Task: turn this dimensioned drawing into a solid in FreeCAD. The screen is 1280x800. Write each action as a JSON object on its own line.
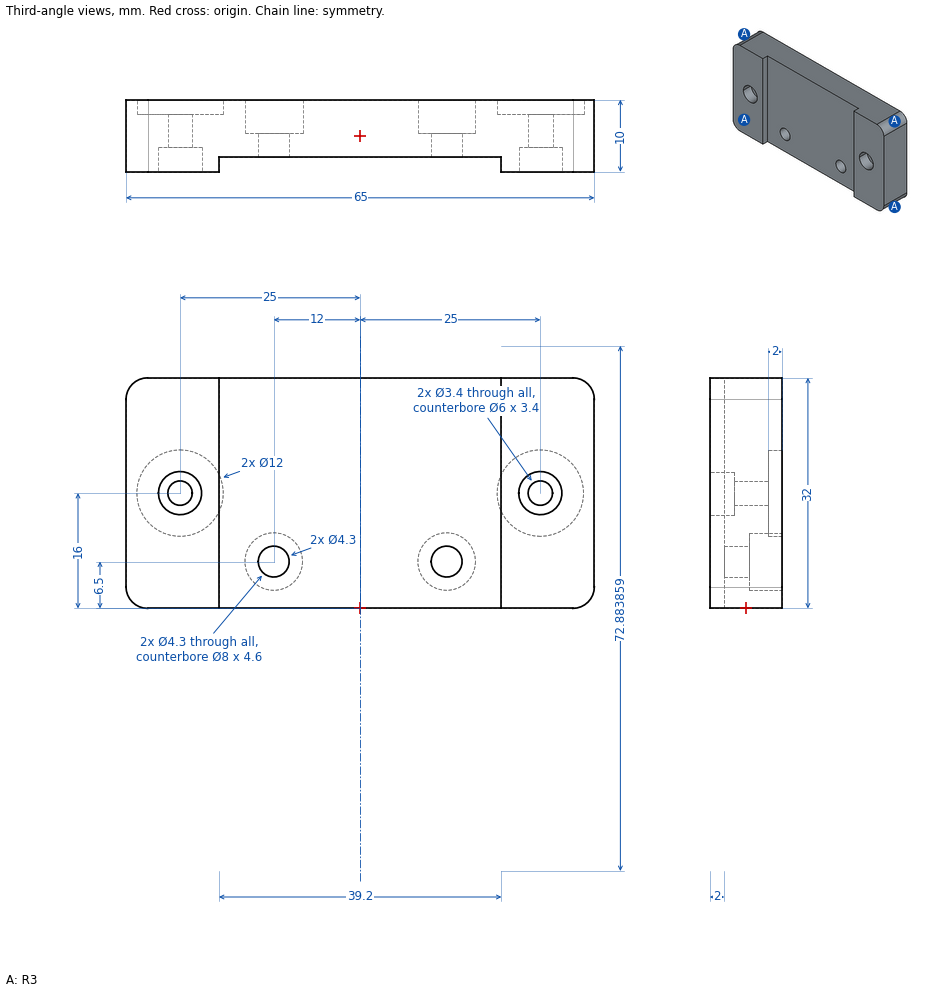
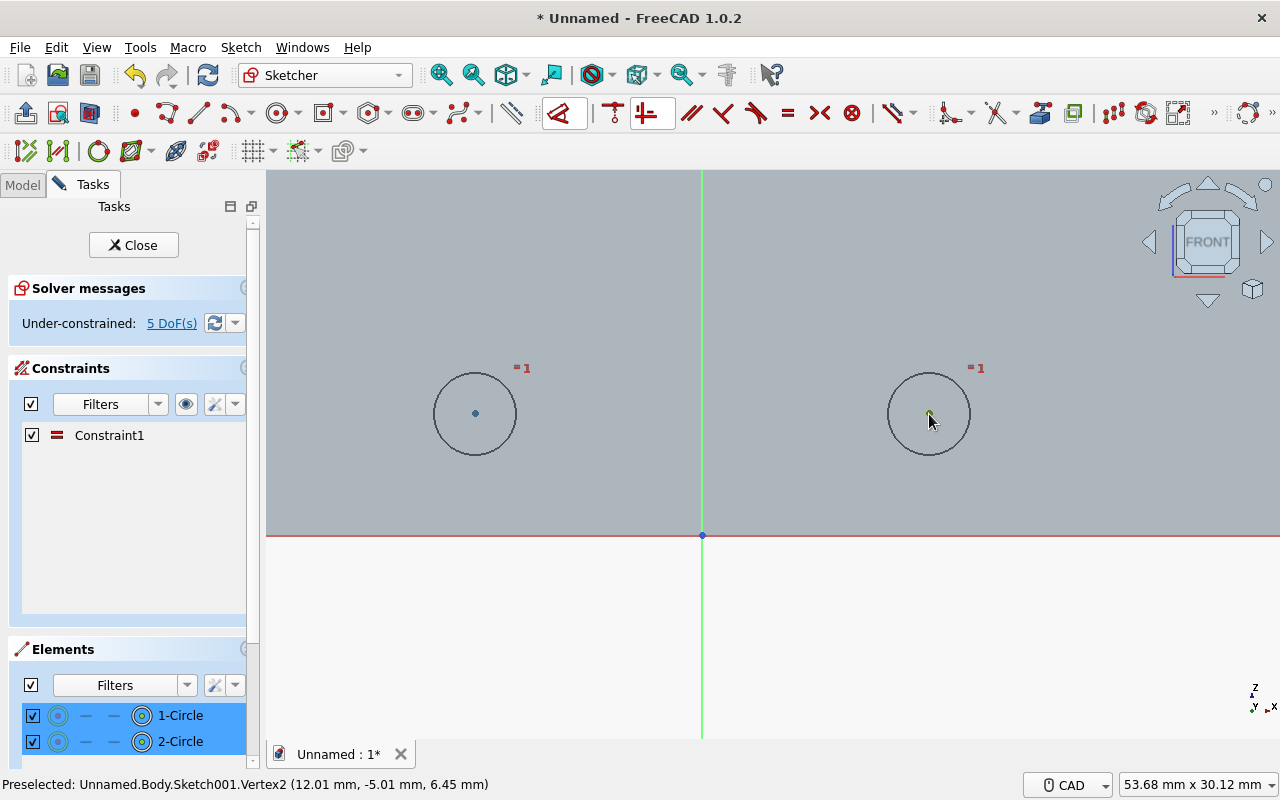
{"action": "left_click", "coordinate": [702, 674]}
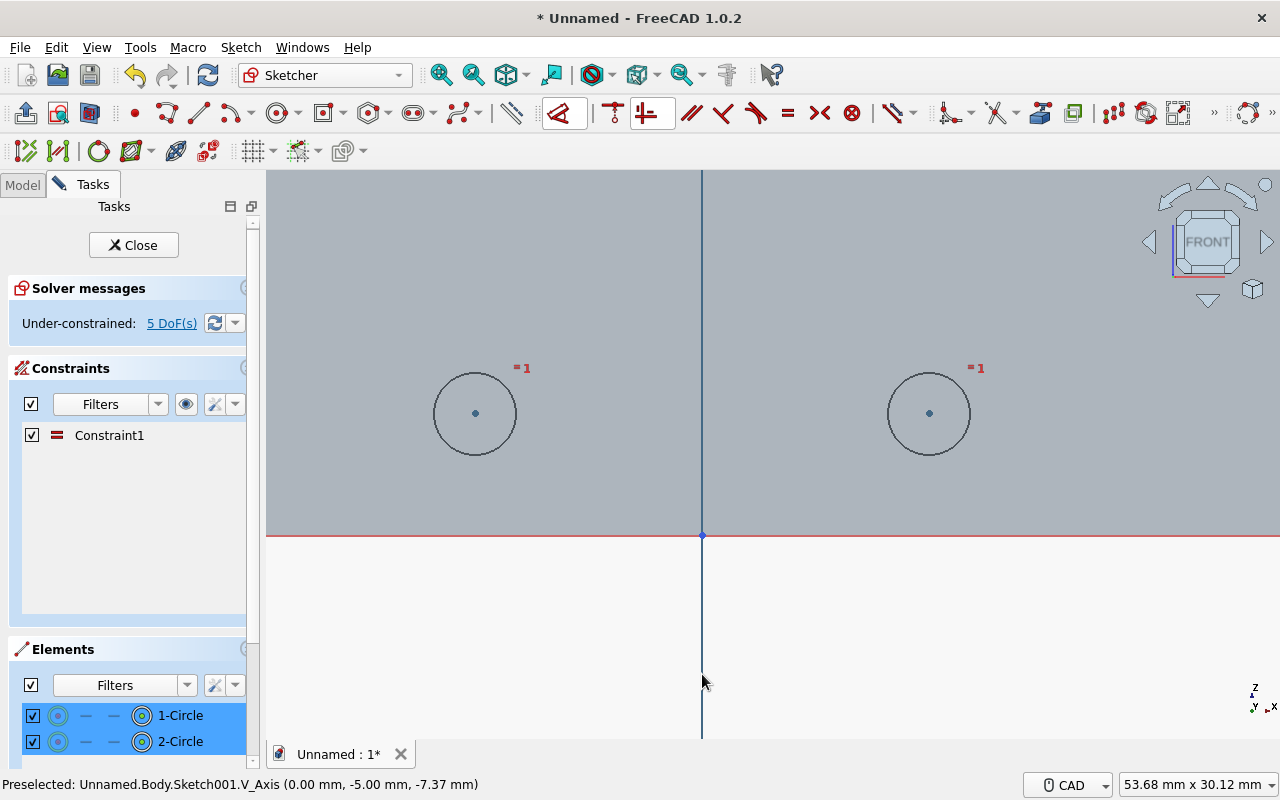
{"action": "left_click", "coordinate": [820, 114]}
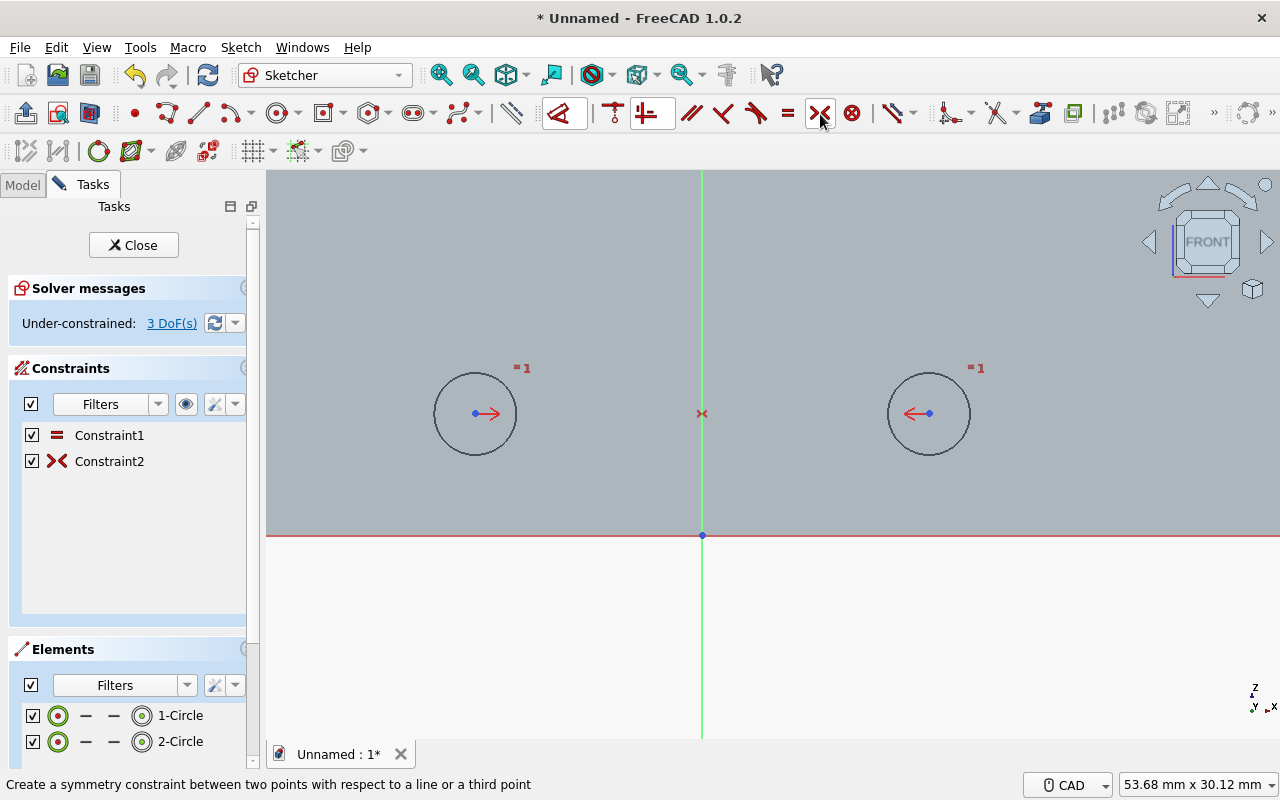
{"action": "left_click", "coordinate": [504, 385]}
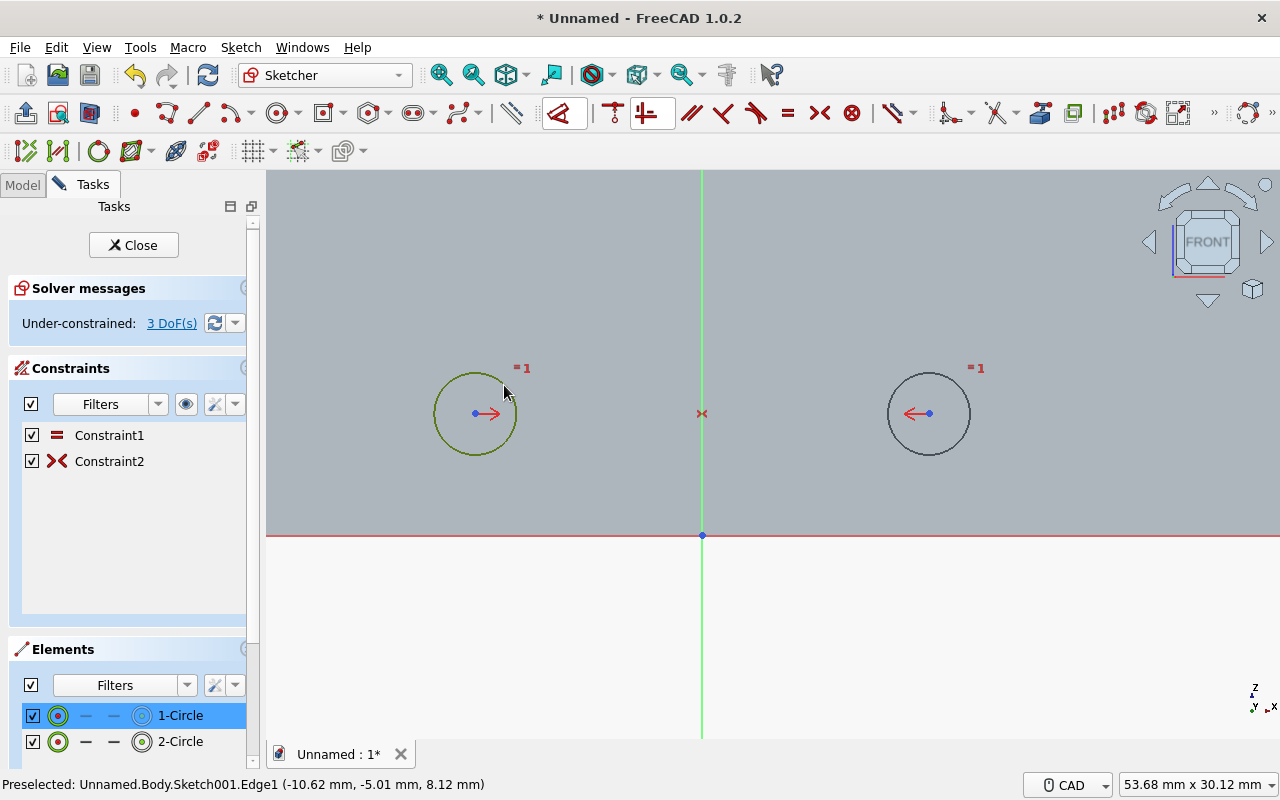
{"action": "key", "text": "k o"}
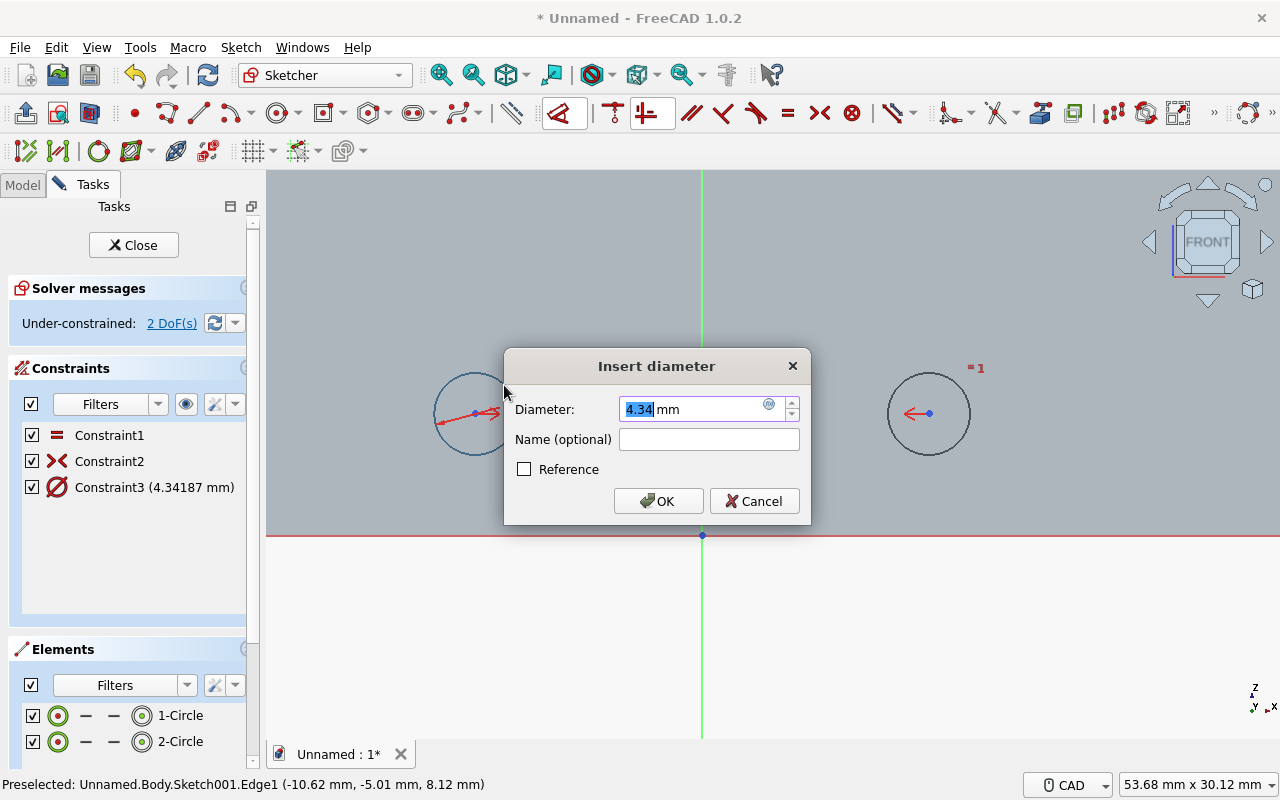
{"action": "type", "text": "4.3"}
{"action": "key", "text": "Return"}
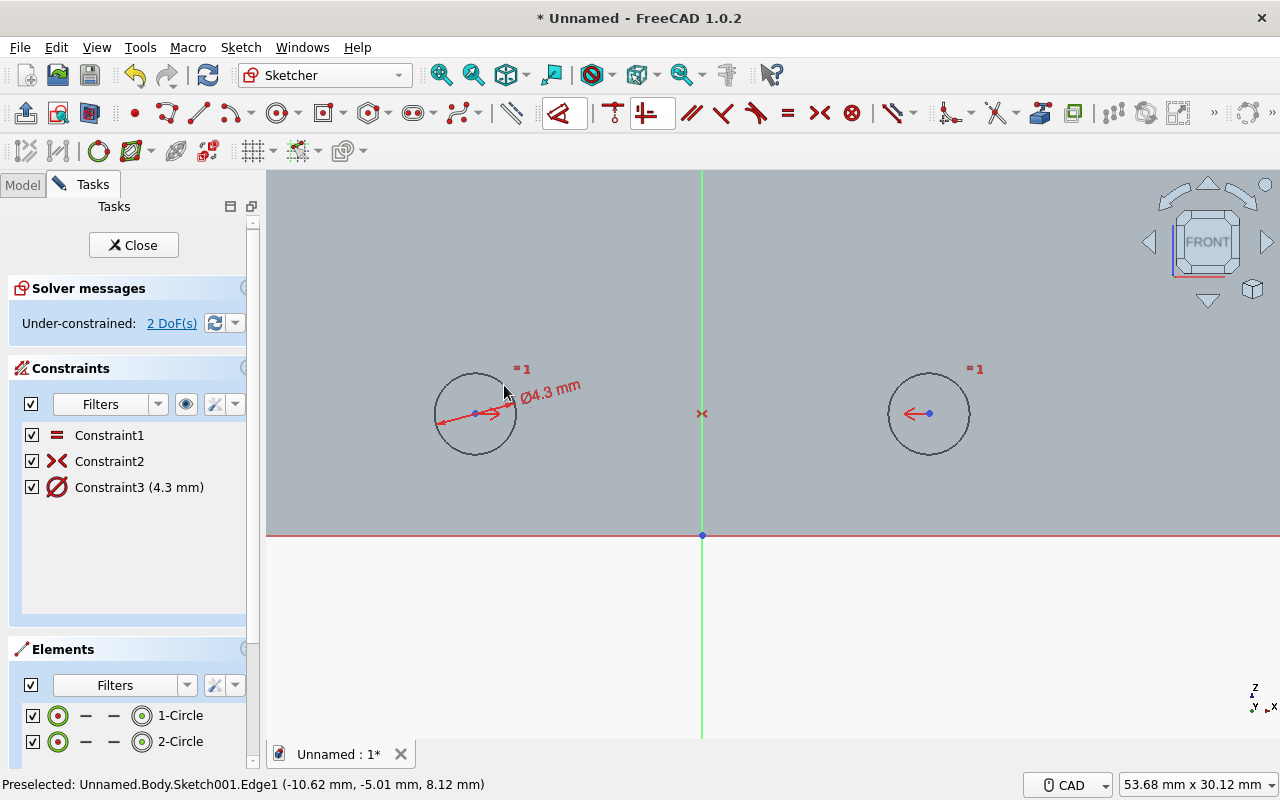
{"action": "left_click", "coordinate": [475, 414]}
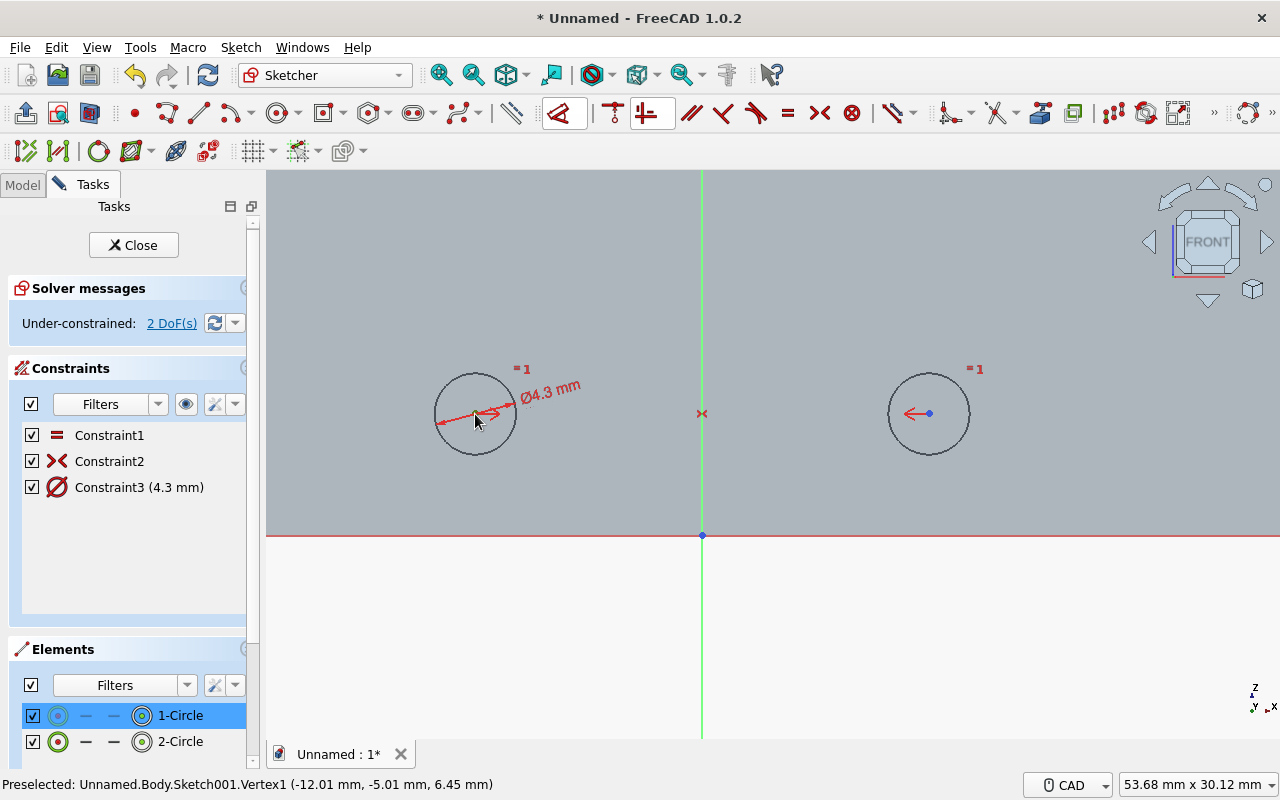
{"action": "key", "text": "l"}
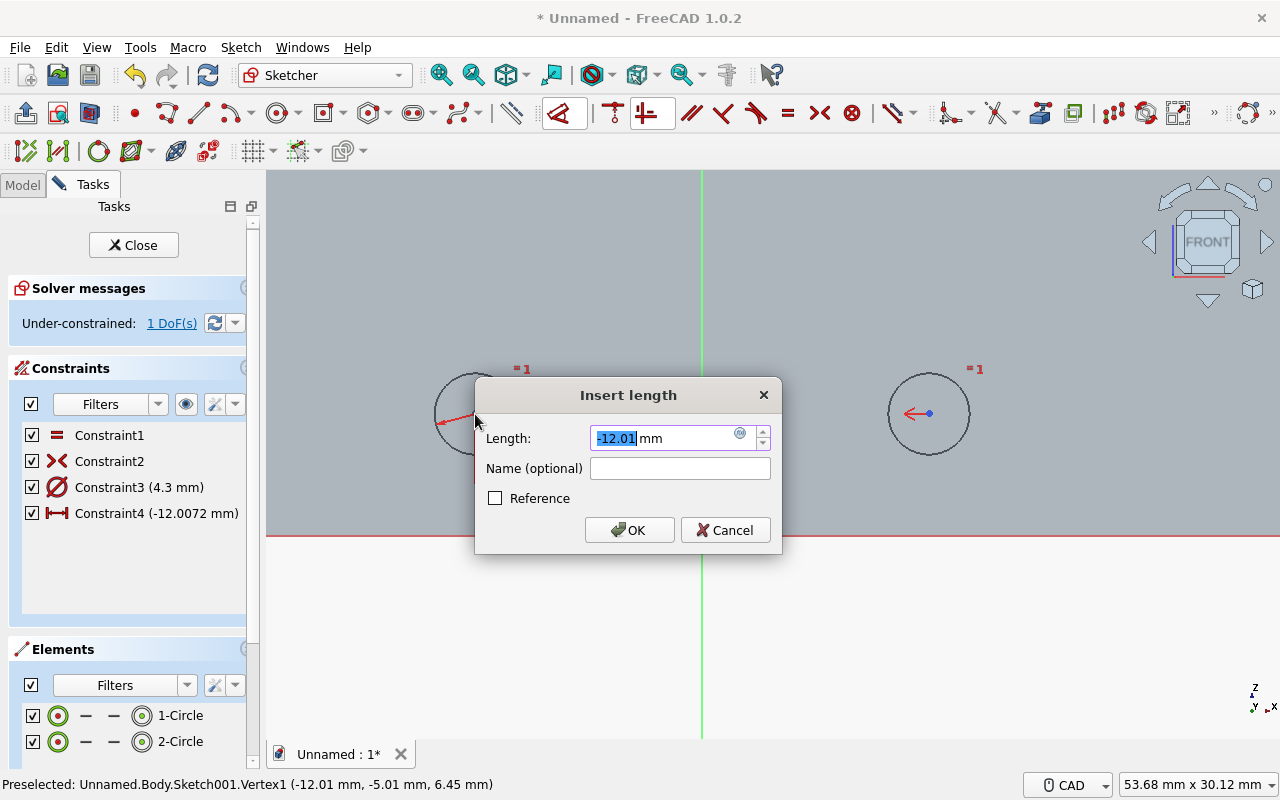
{"action": "type", "text": "-12"}
{"action": "key", "text": "Return"}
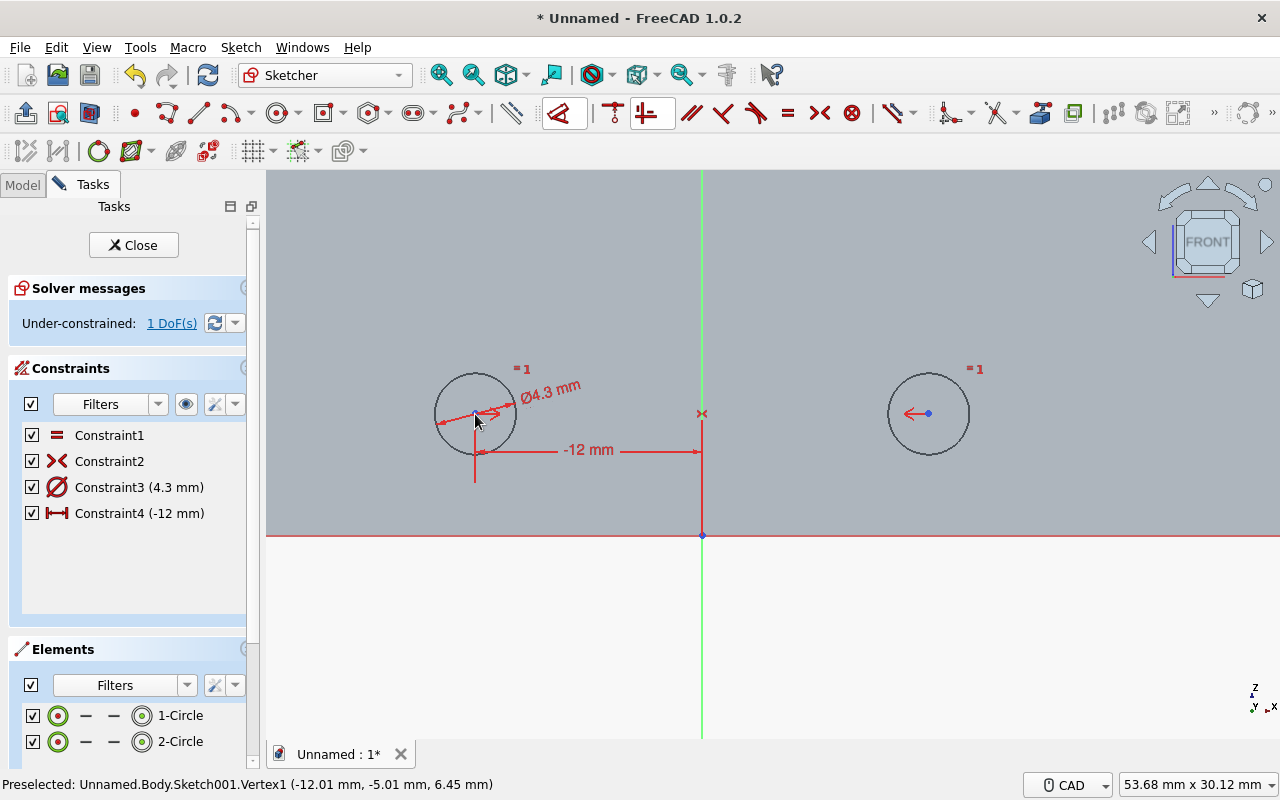
{"action": "left_click", "coordinate": [475, 414]}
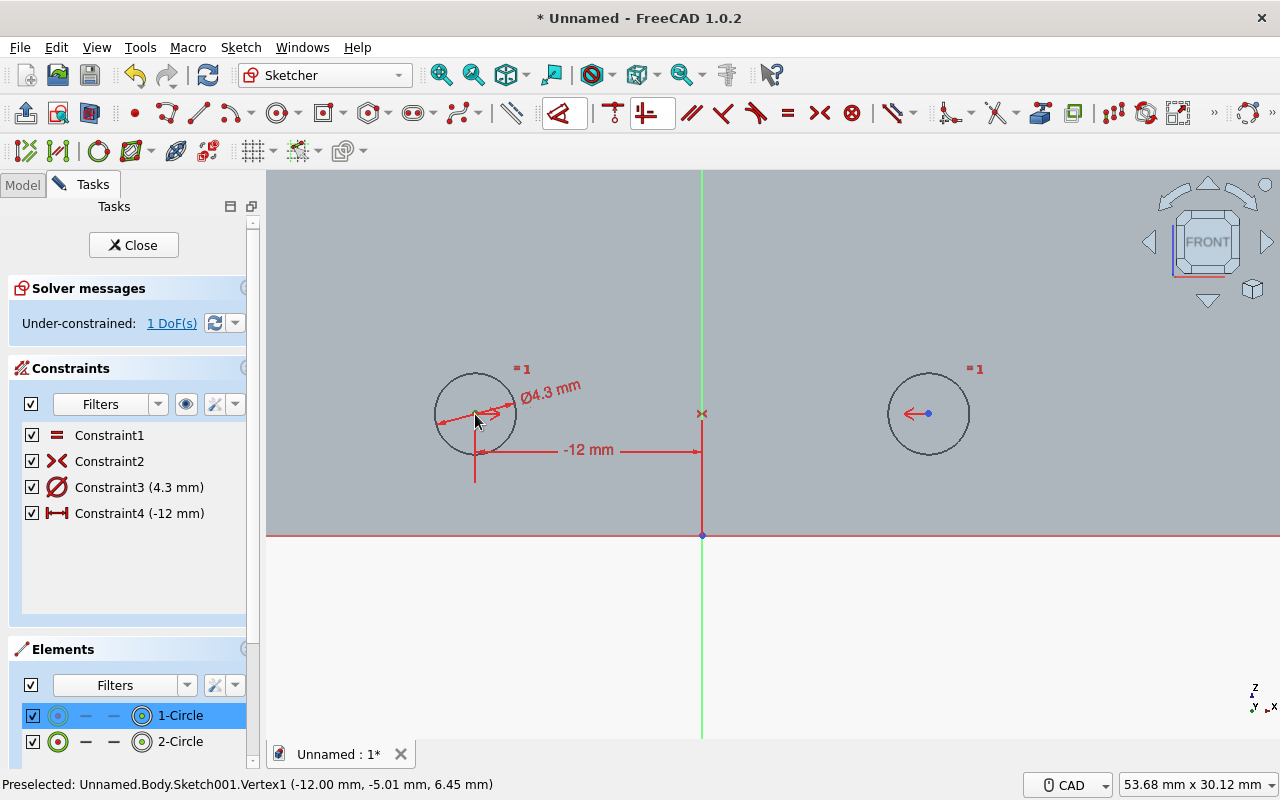
{"action": "key", "text": "i"}